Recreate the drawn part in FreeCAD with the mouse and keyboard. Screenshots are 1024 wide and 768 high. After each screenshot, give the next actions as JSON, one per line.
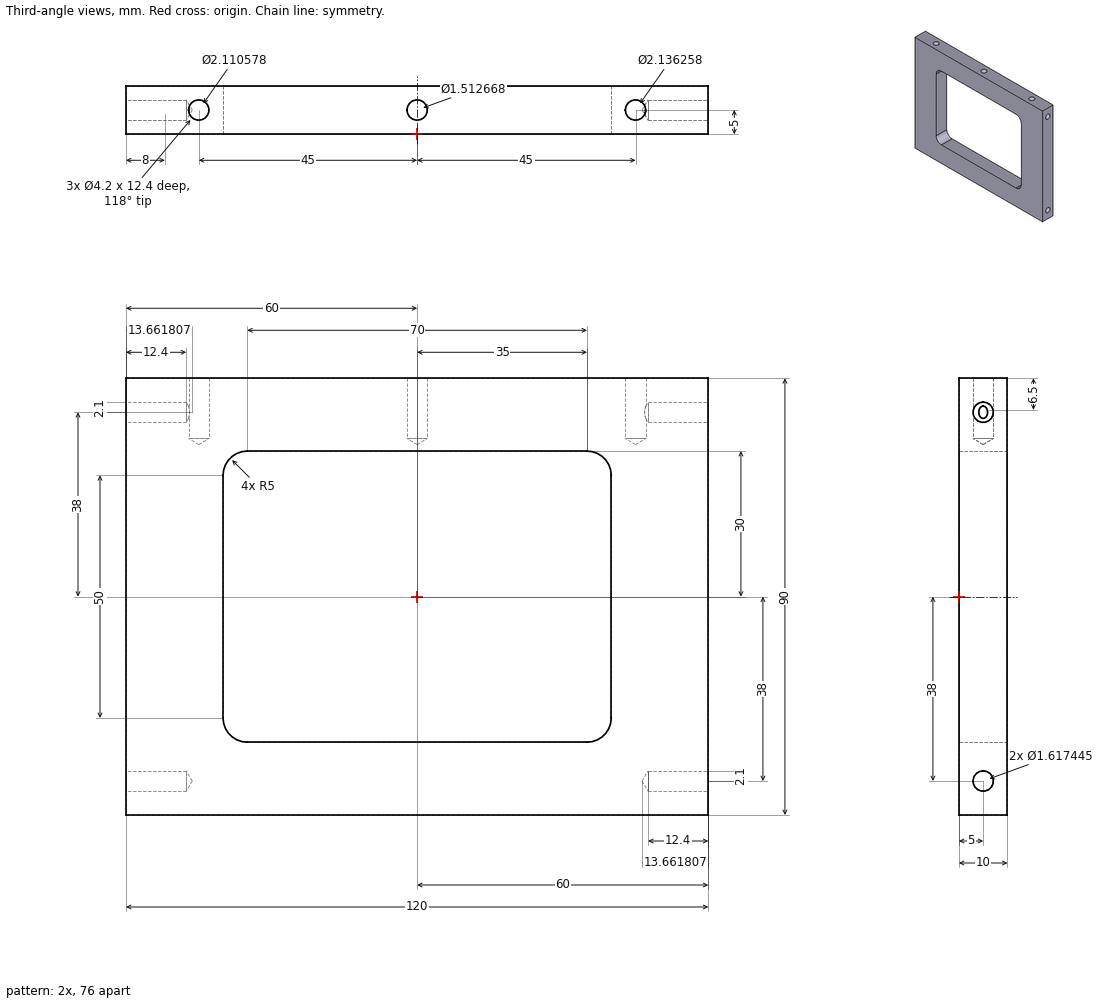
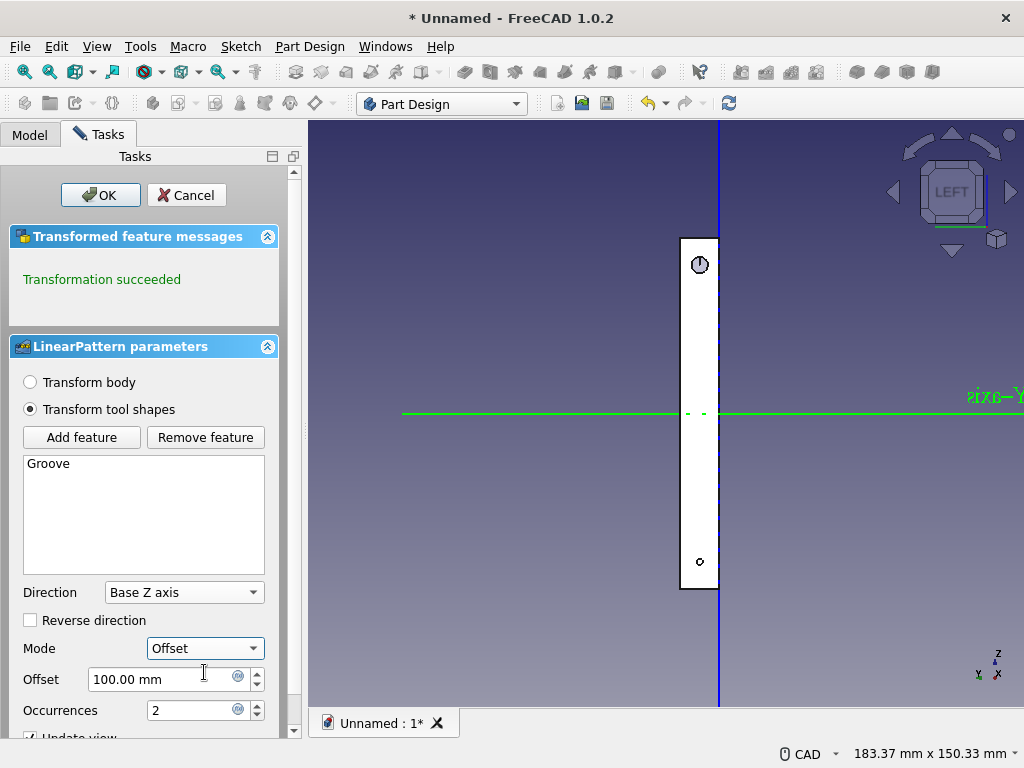
{"action": "triple_click", "coordinate": [170, 680]}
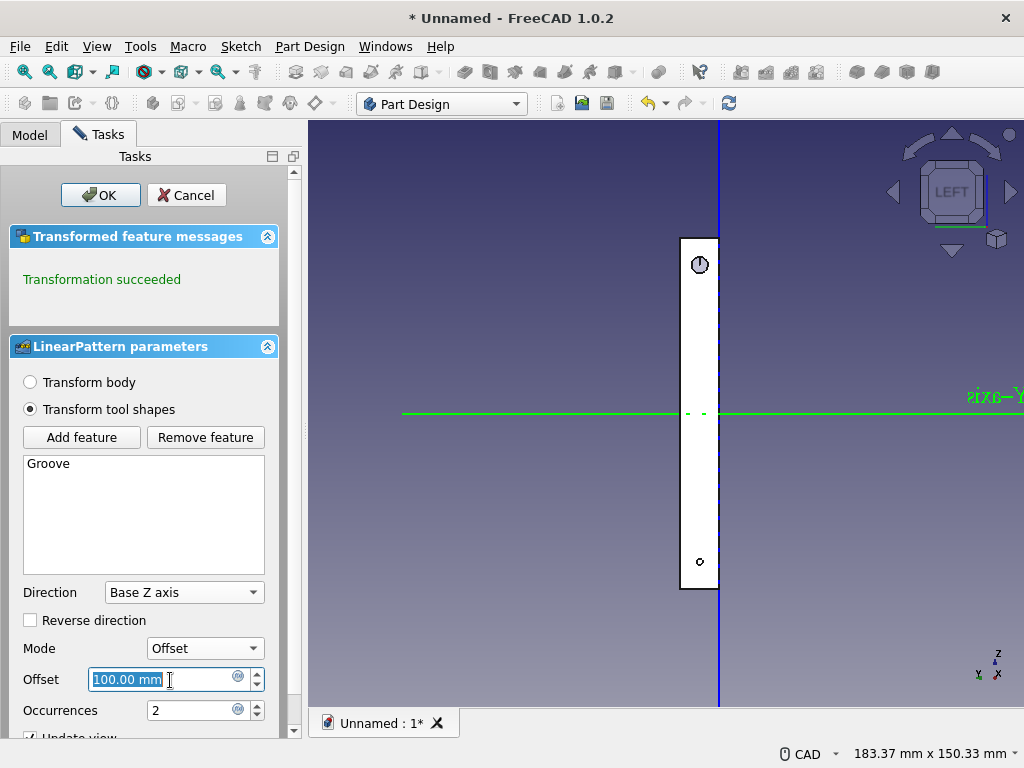
{"action": "type", "text": "76"}
{"action": "key", "text": "Tab"}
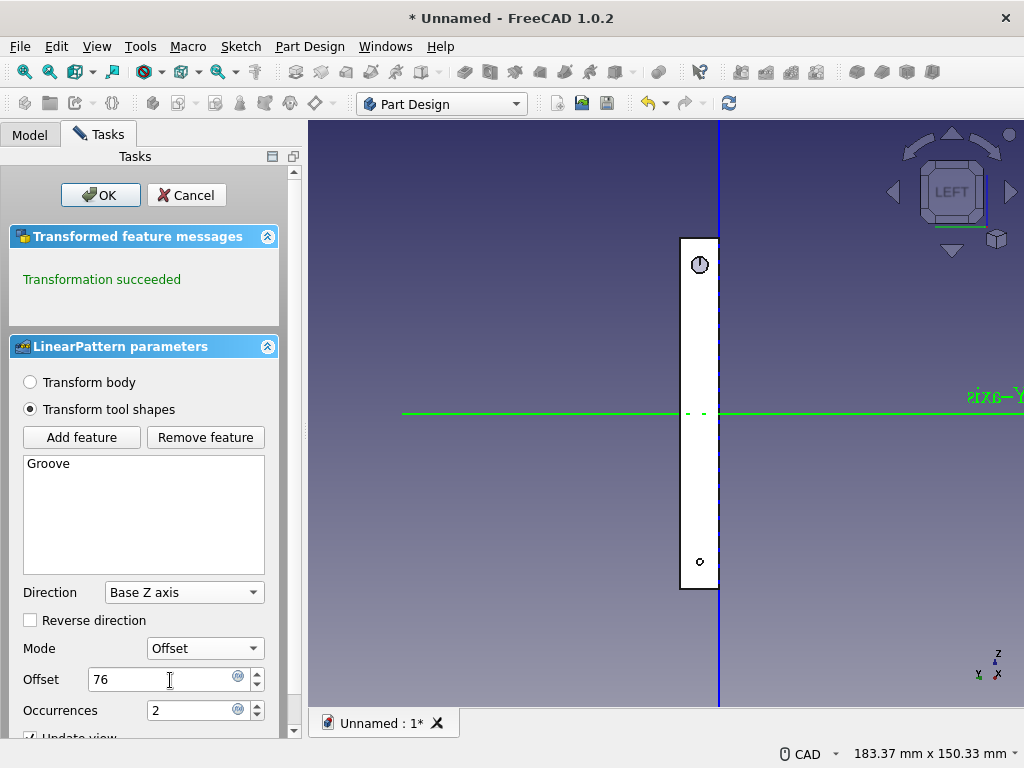
{"action": "triple_click", "coordinate": [199, 710]}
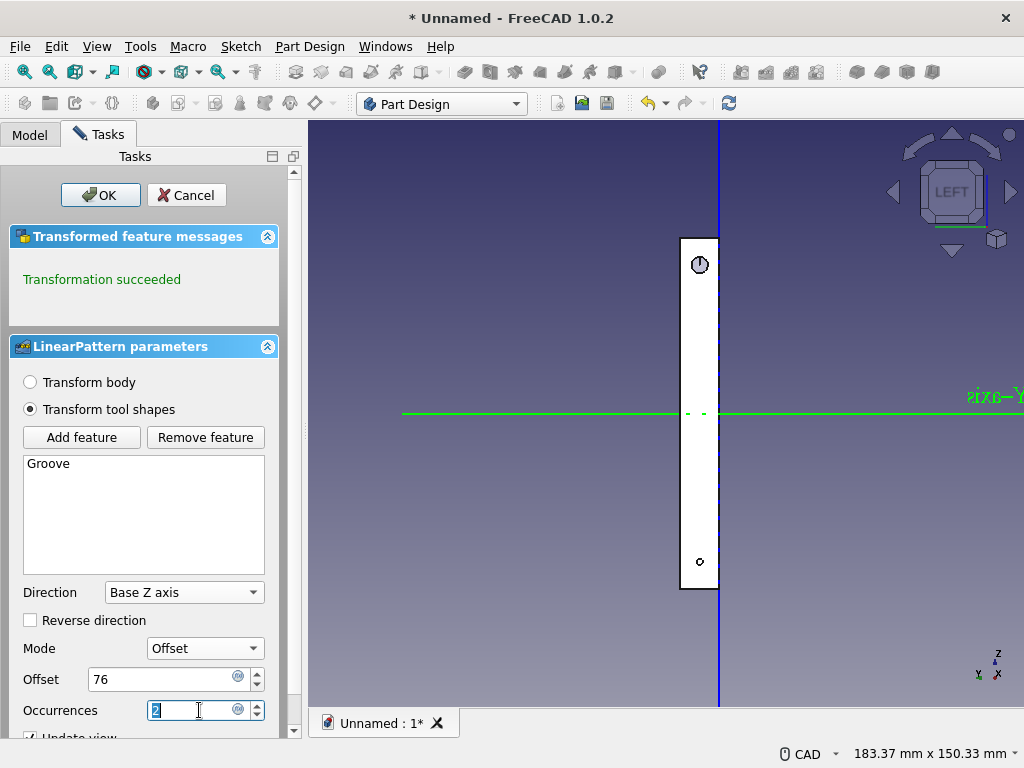
{"action": "type", "text": "2"}
{"action": "key", "text": "Tab"}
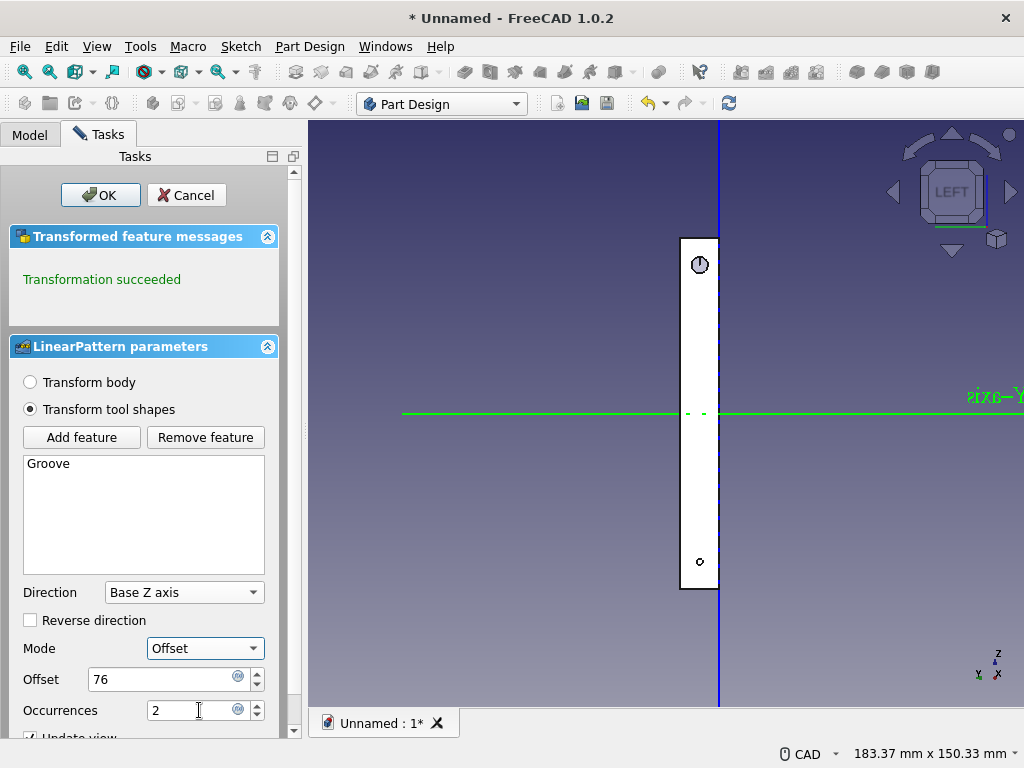
{"action": "left_click", "coordinate": [31, 620]}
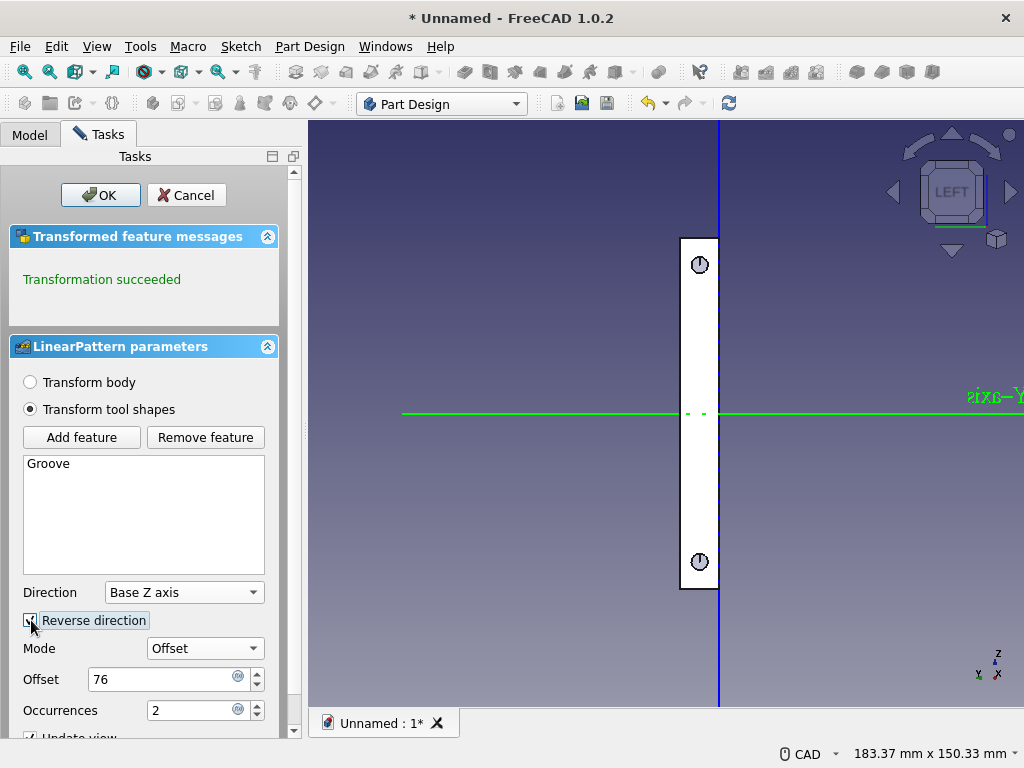
{"action": "left_click", "coordinate": [101, 195]}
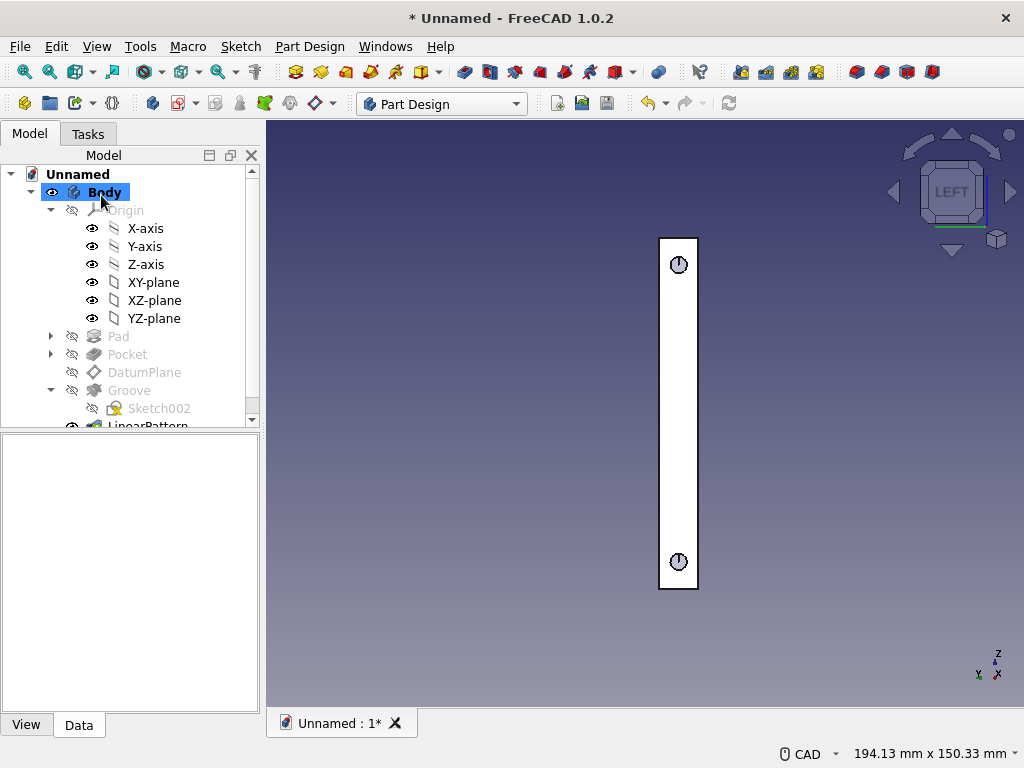
{"action": "left_click", "coordinate": [117, 390]}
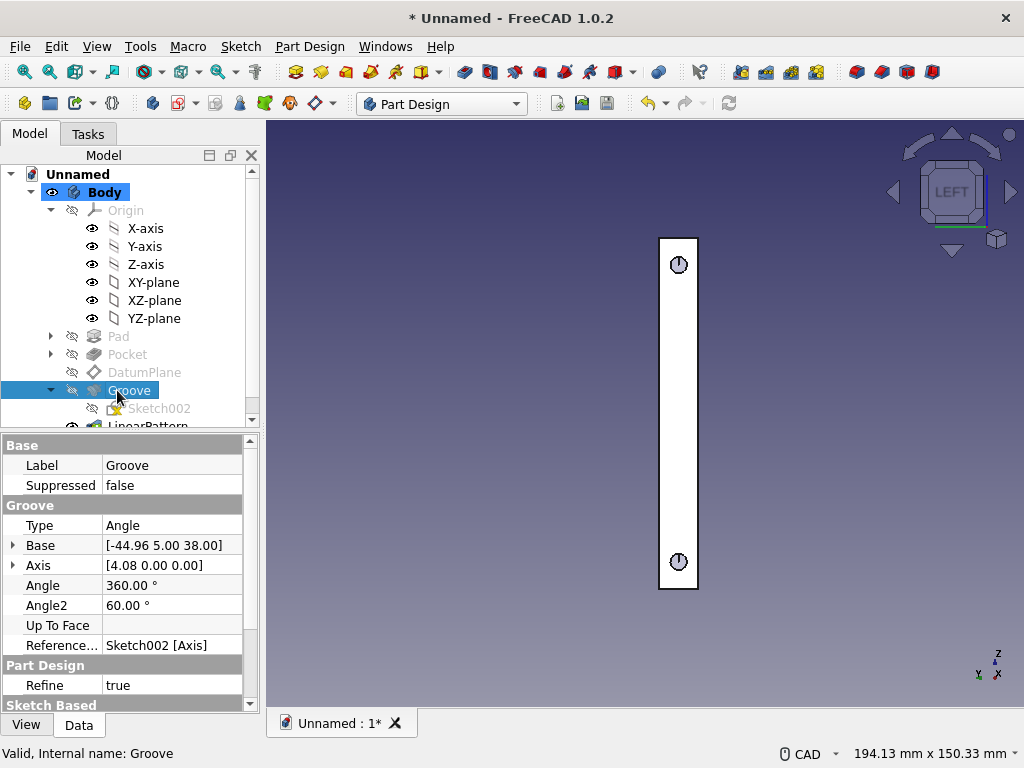
{"action": "left_click", "coordinate": [741, 72]}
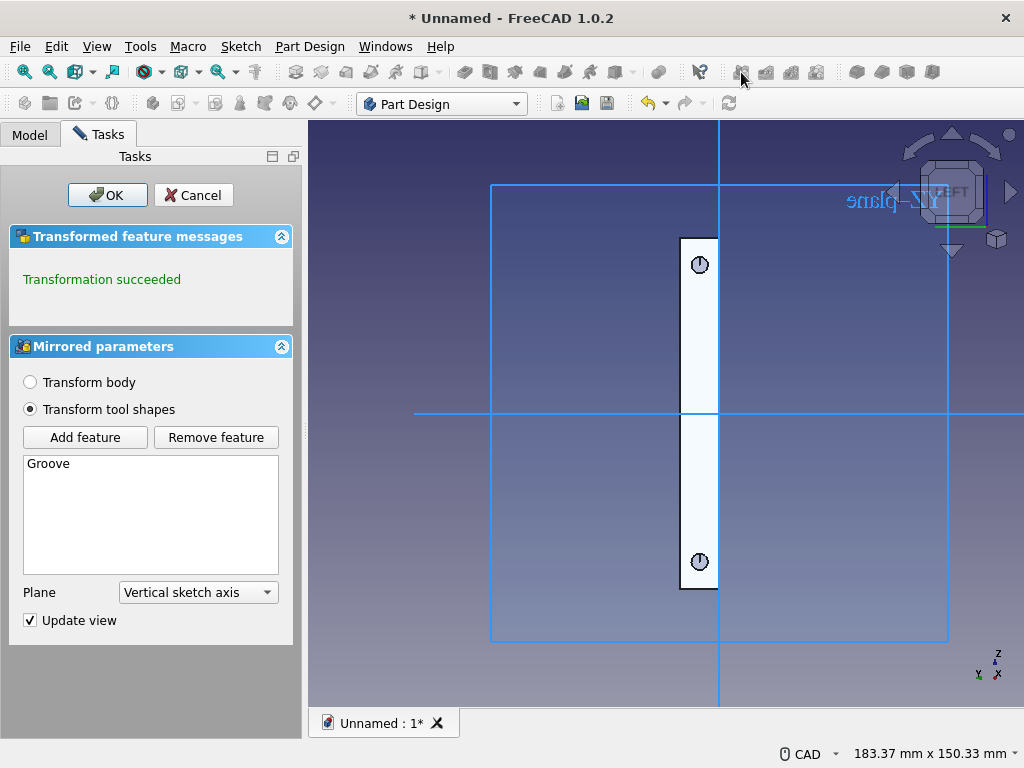
{"action": "left_click", "coordinate": [199, 592]}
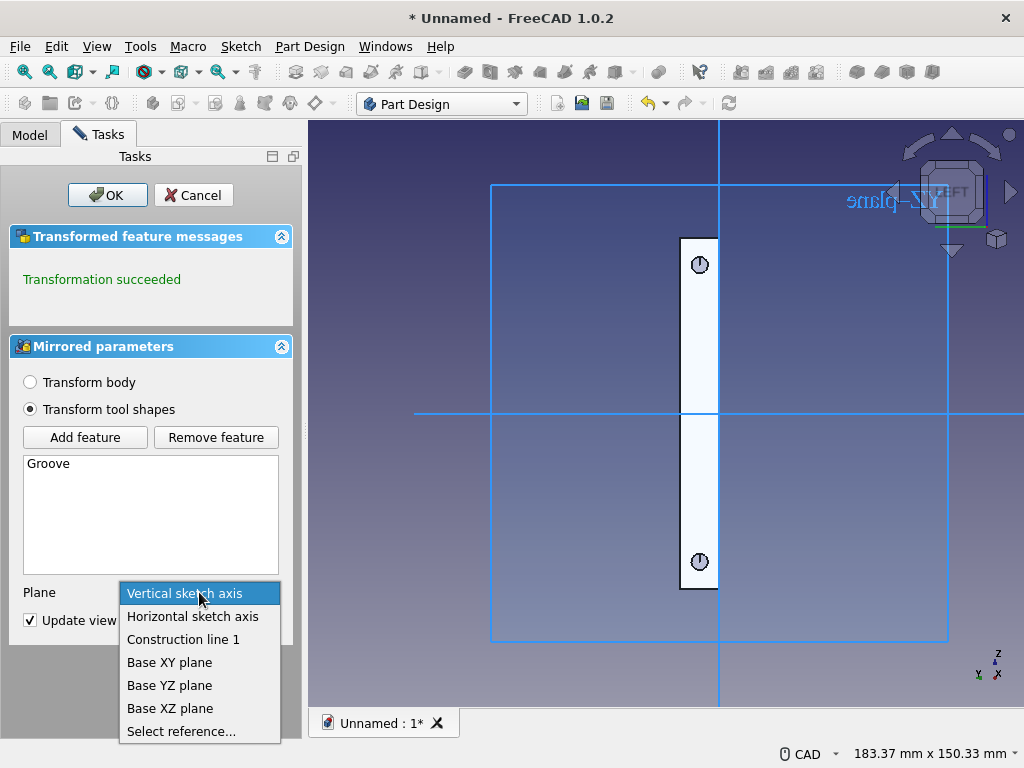
{"action": "left_click", "coordinate": [198, 686]}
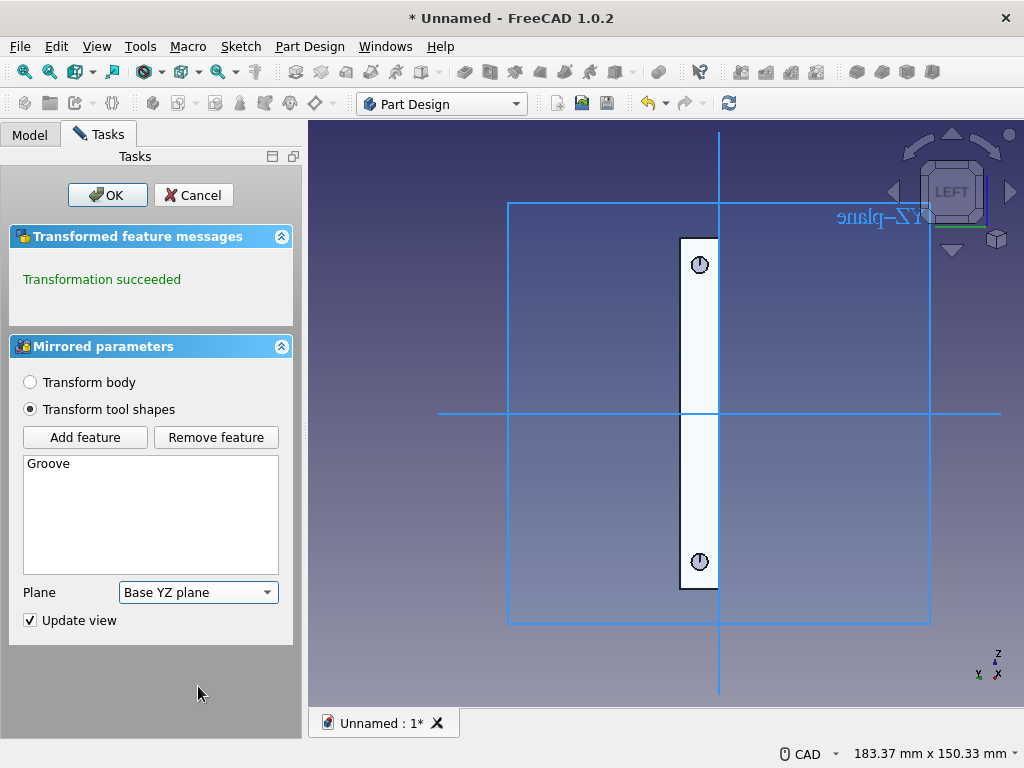
{"action": "left_click", "coordinate": [108, 195]}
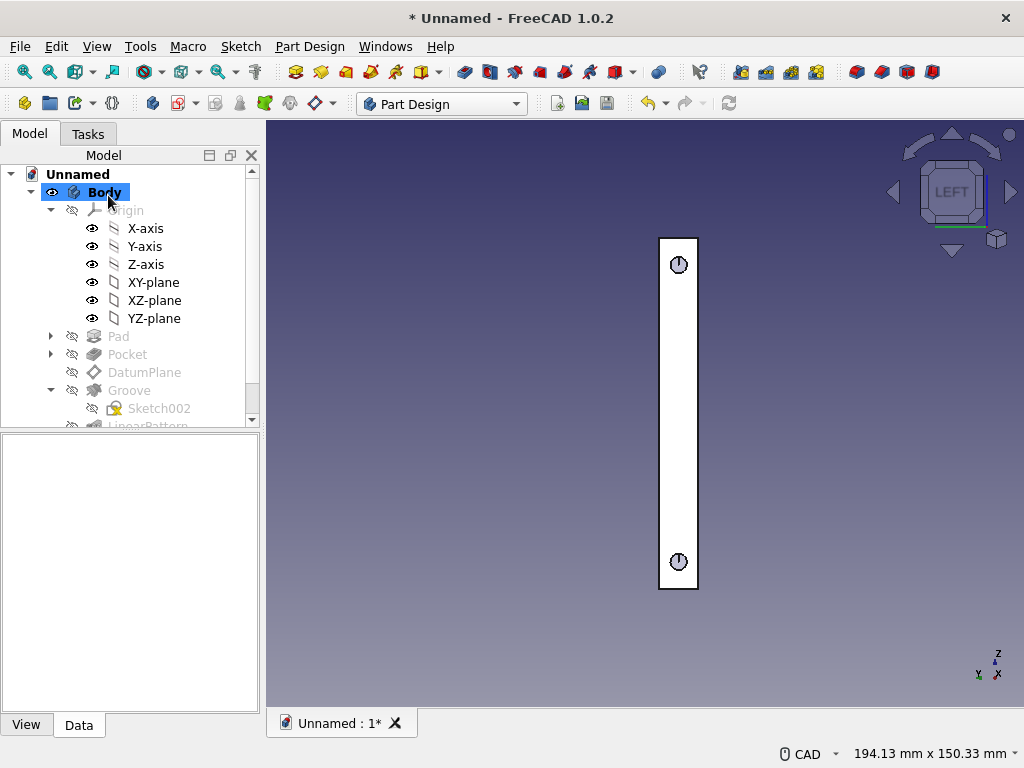
{"action": "left_click", "coordinate": [137, 300]}